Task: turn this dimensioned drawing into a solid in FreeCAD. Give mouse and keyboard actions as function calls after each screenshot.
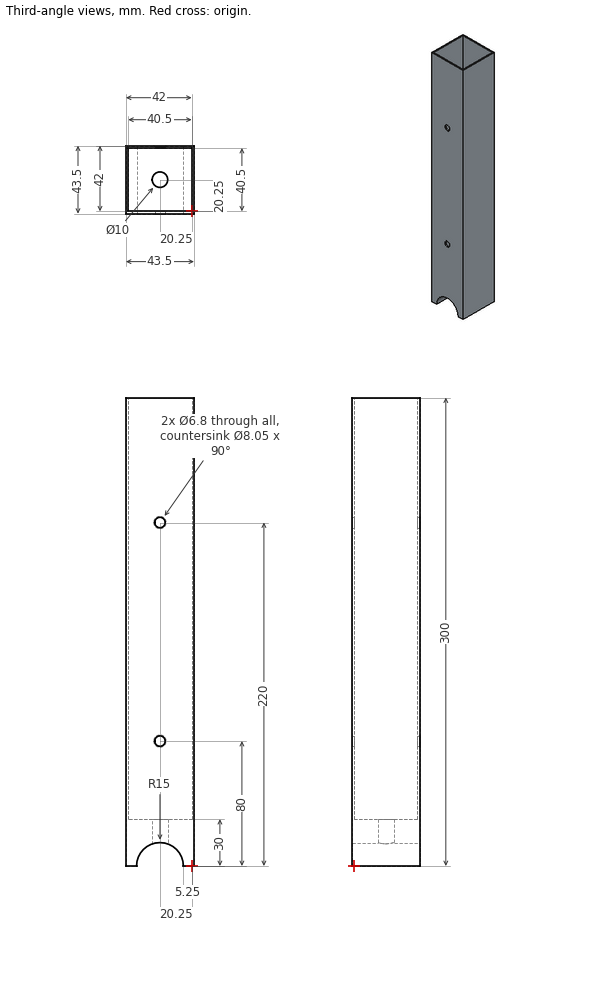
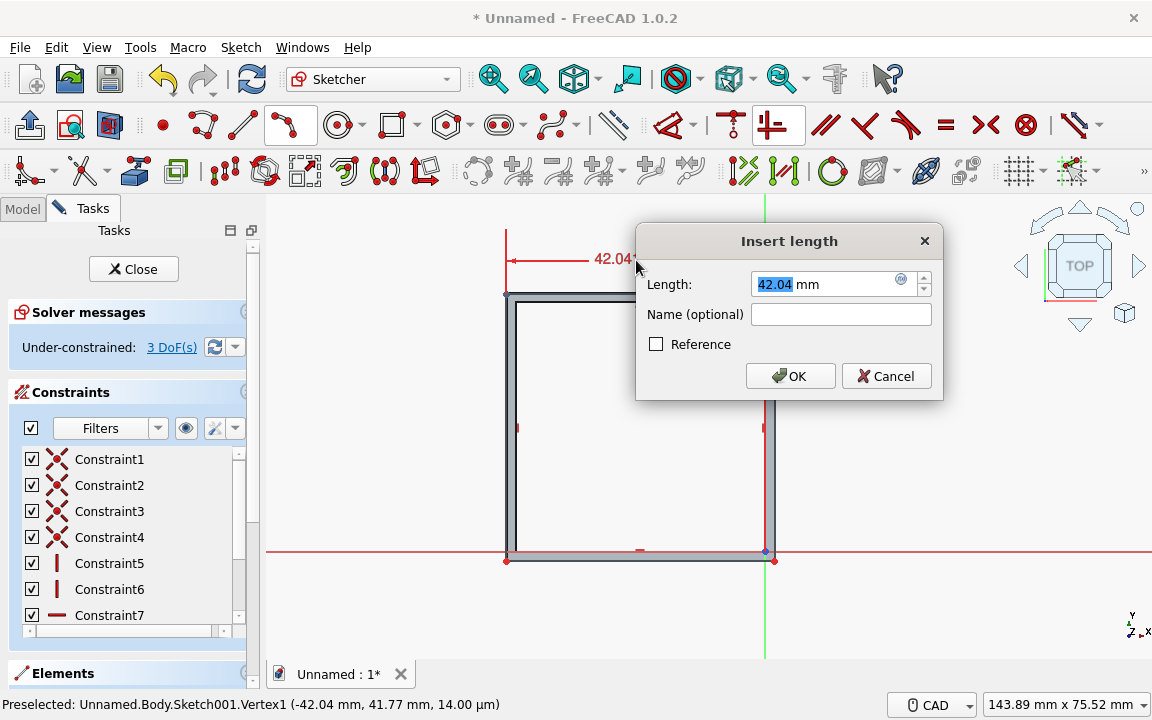
text(42)
key(Return)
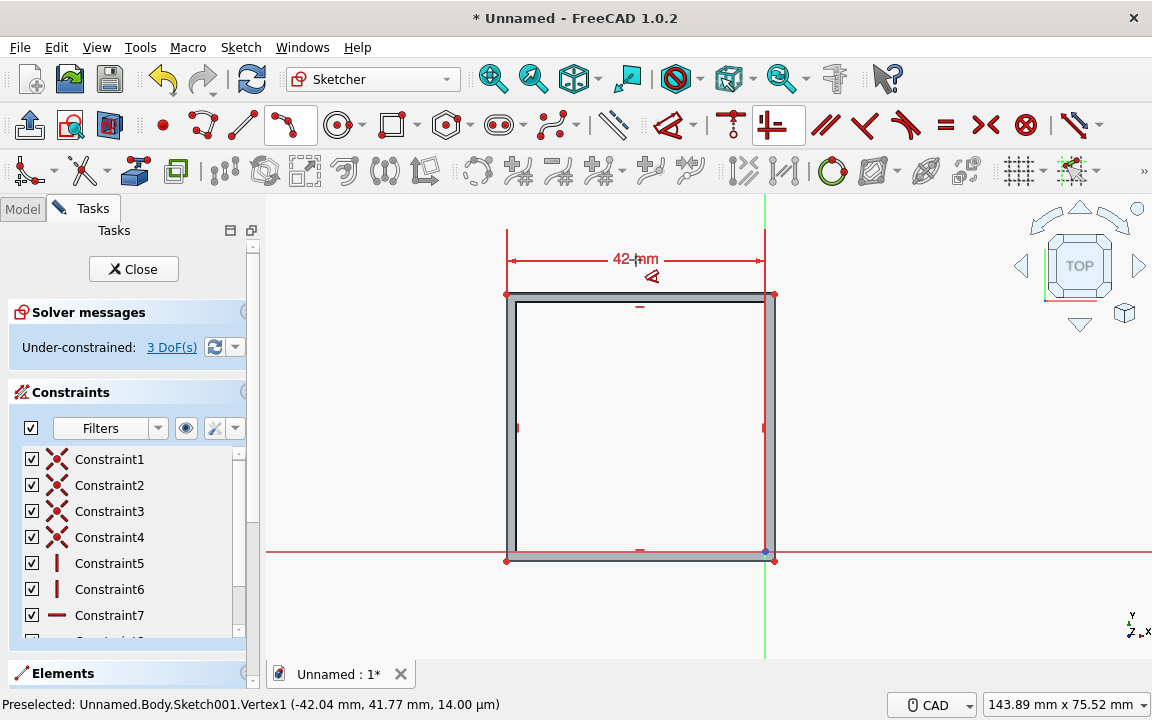
click(507, 294)
click(473, 423)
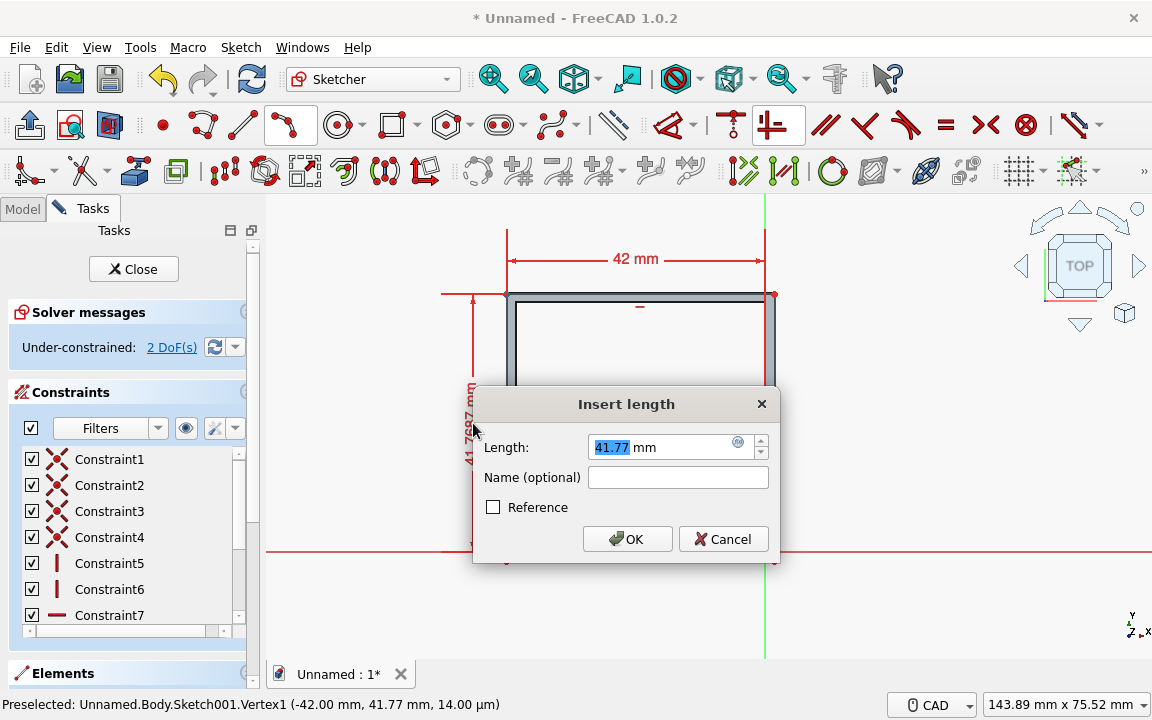
text(42)
key(Return)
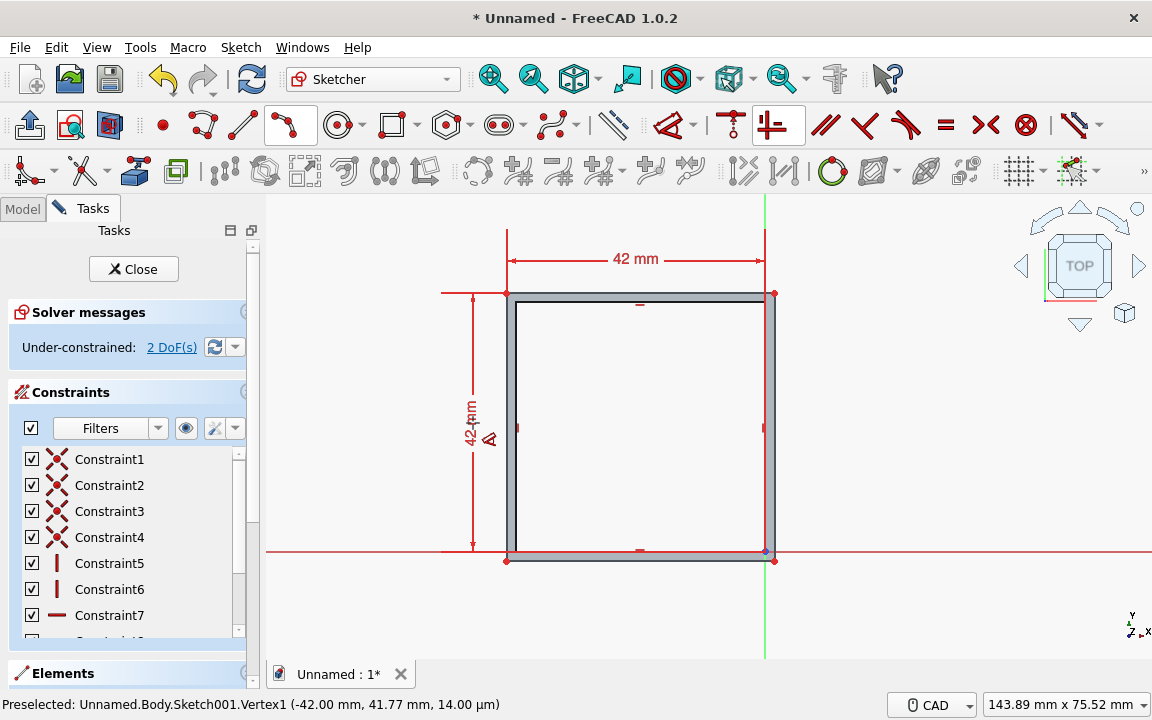
click(507, 374)
click(473, 365)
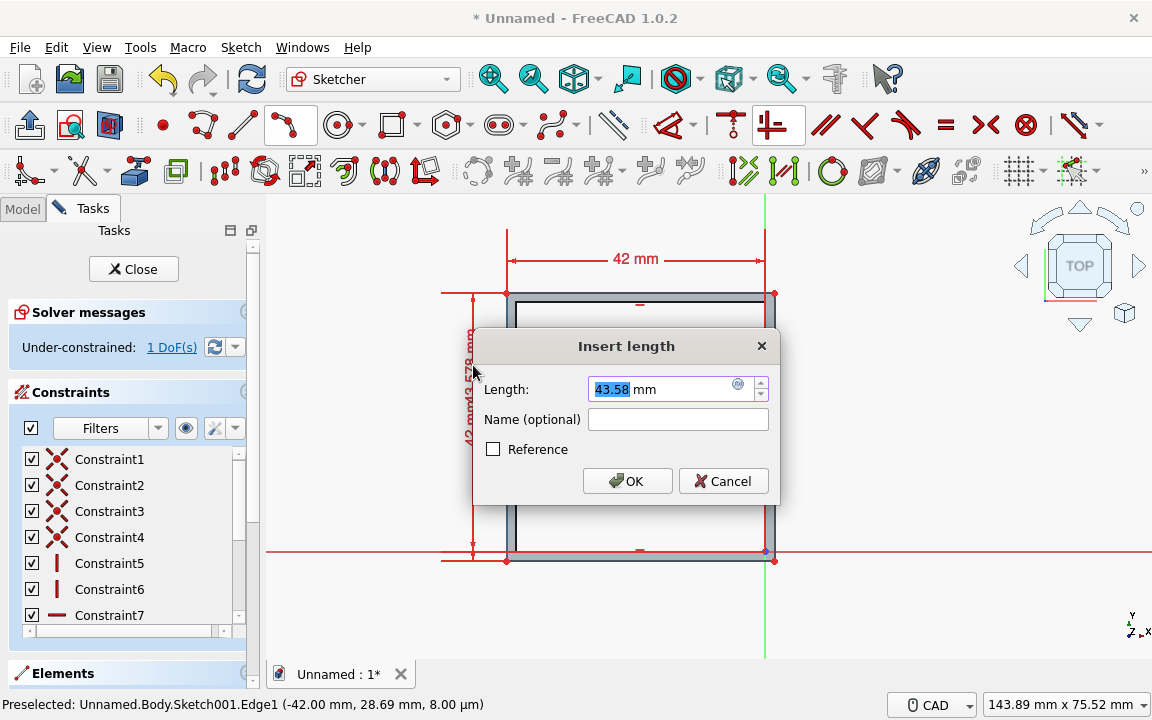
text(43.5)
key(Return)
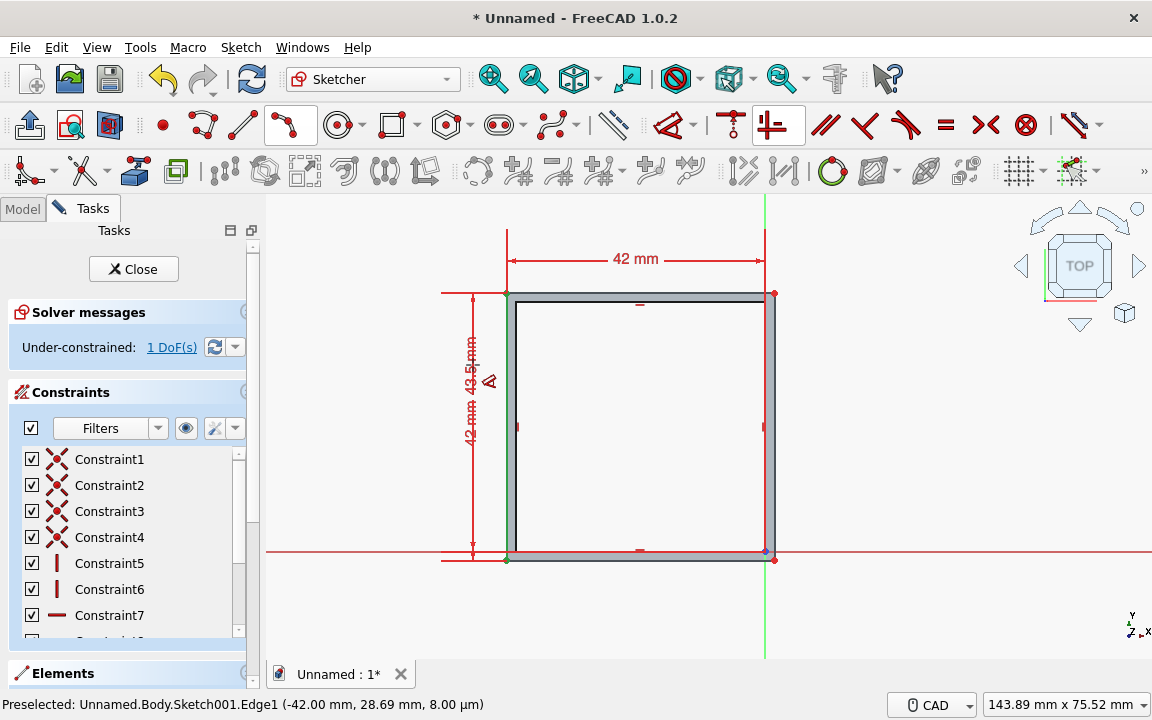
scroll(587, 561, up, 3)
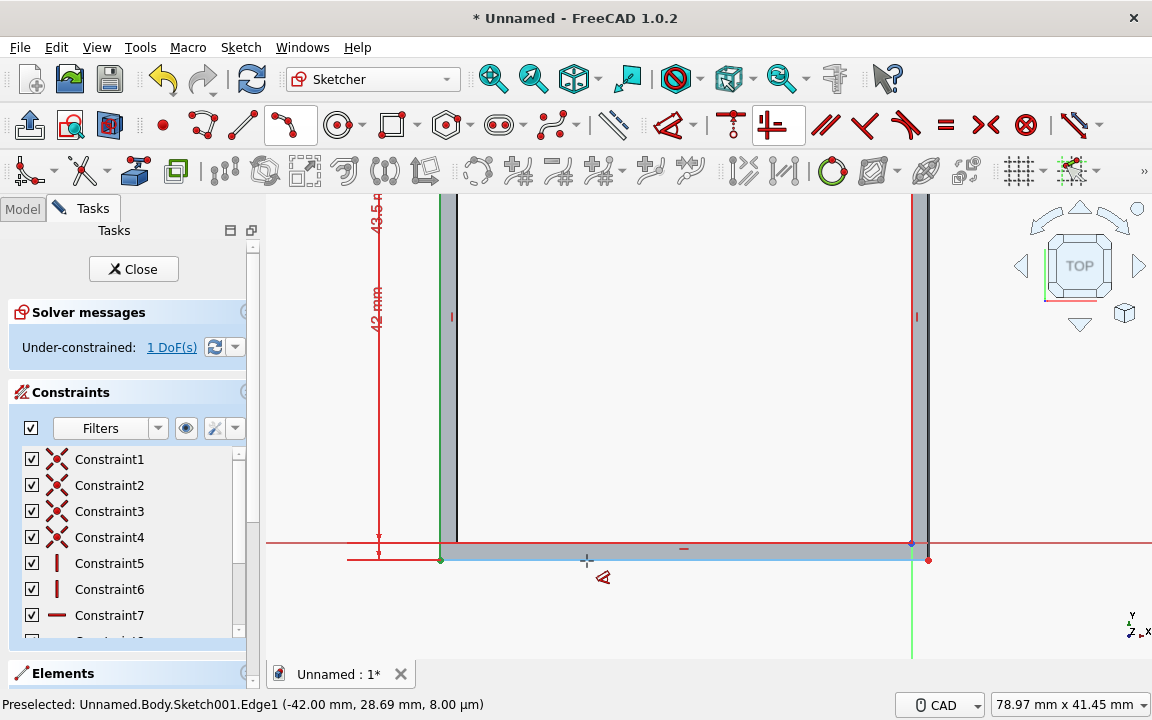
click(587, 560)
click(685, 594)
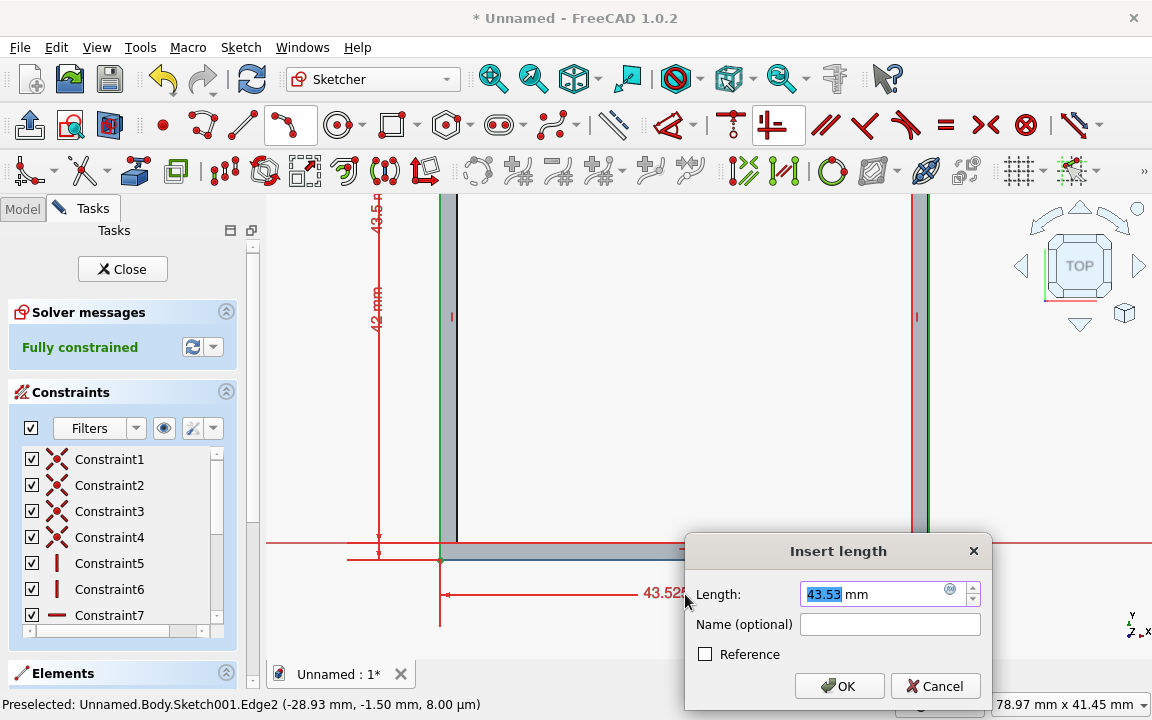
text(43.5)
key(Return)
key(Escape)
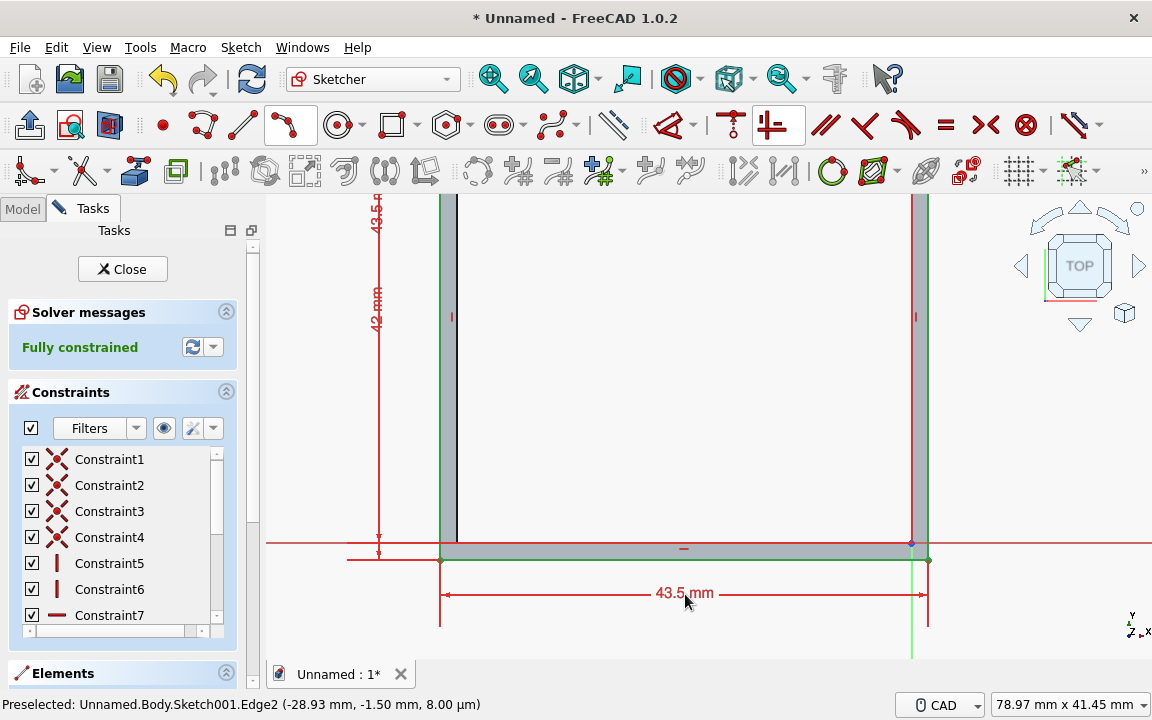
click(123, 269)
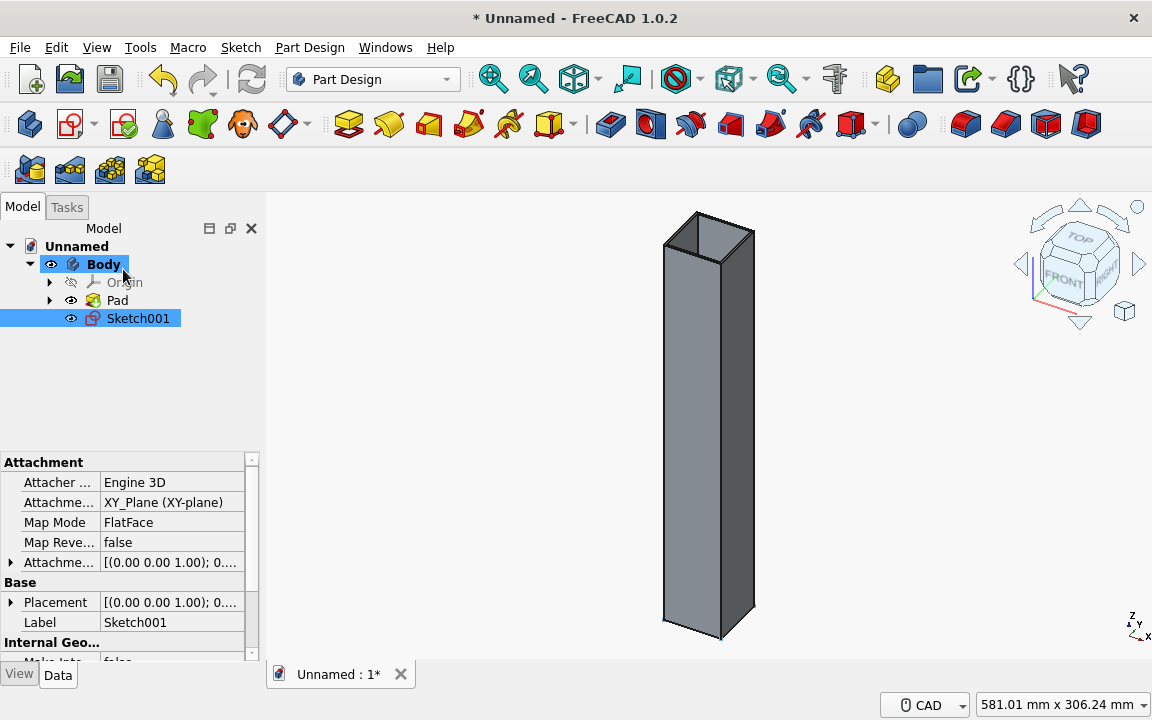
click(350, 124)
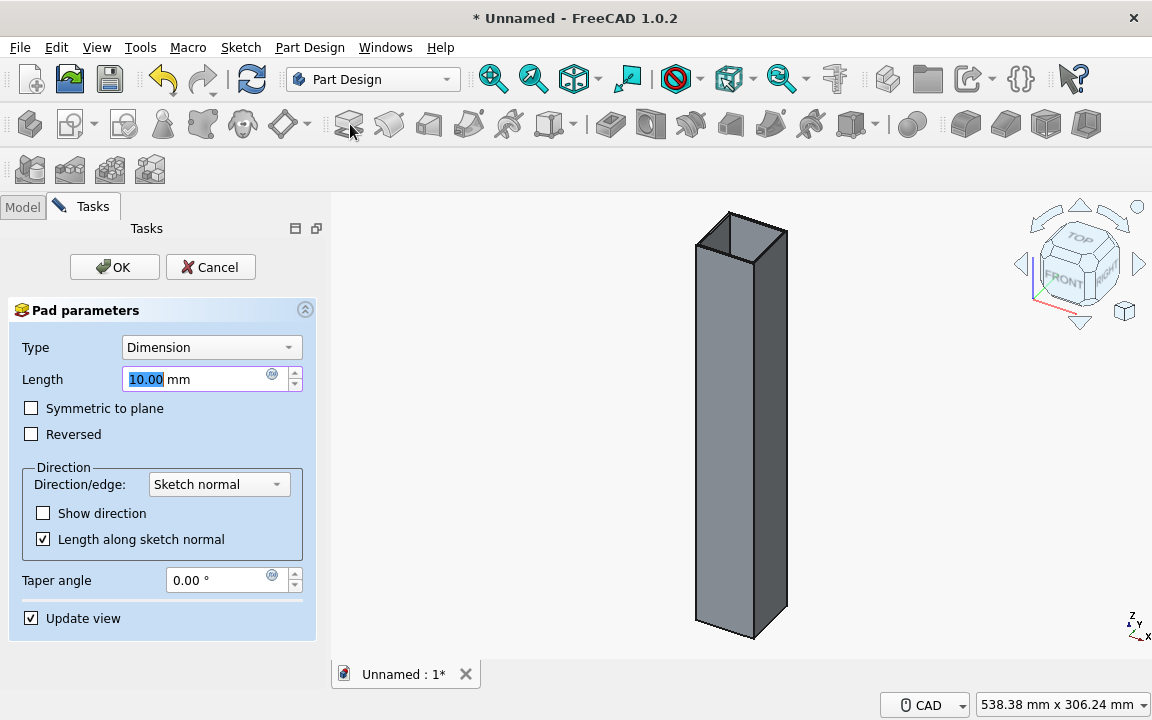
text(30)
key(Tab)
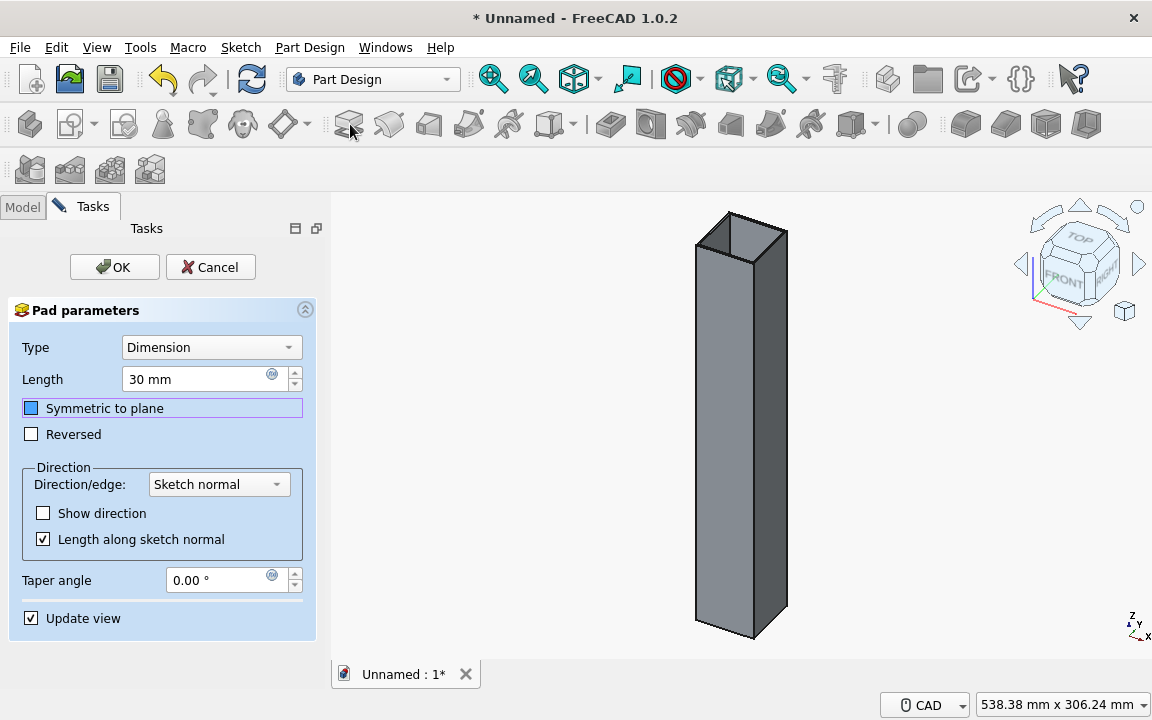
click(115, 267)